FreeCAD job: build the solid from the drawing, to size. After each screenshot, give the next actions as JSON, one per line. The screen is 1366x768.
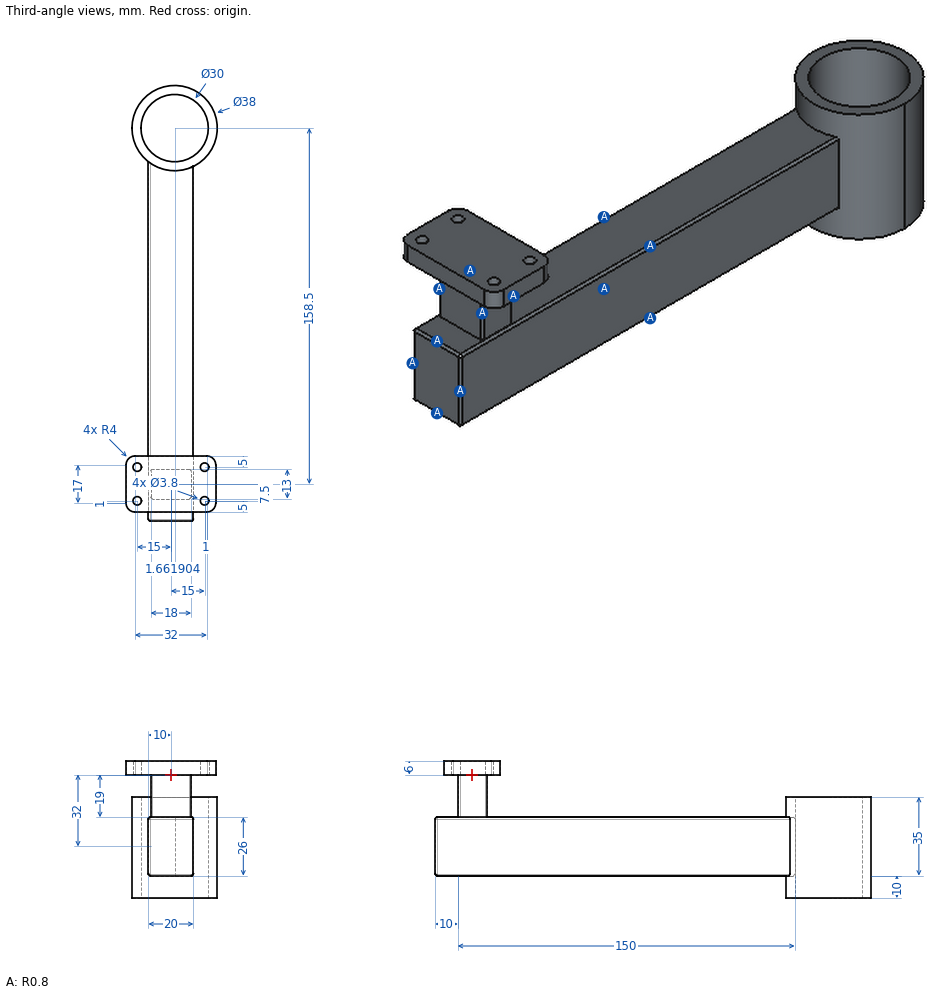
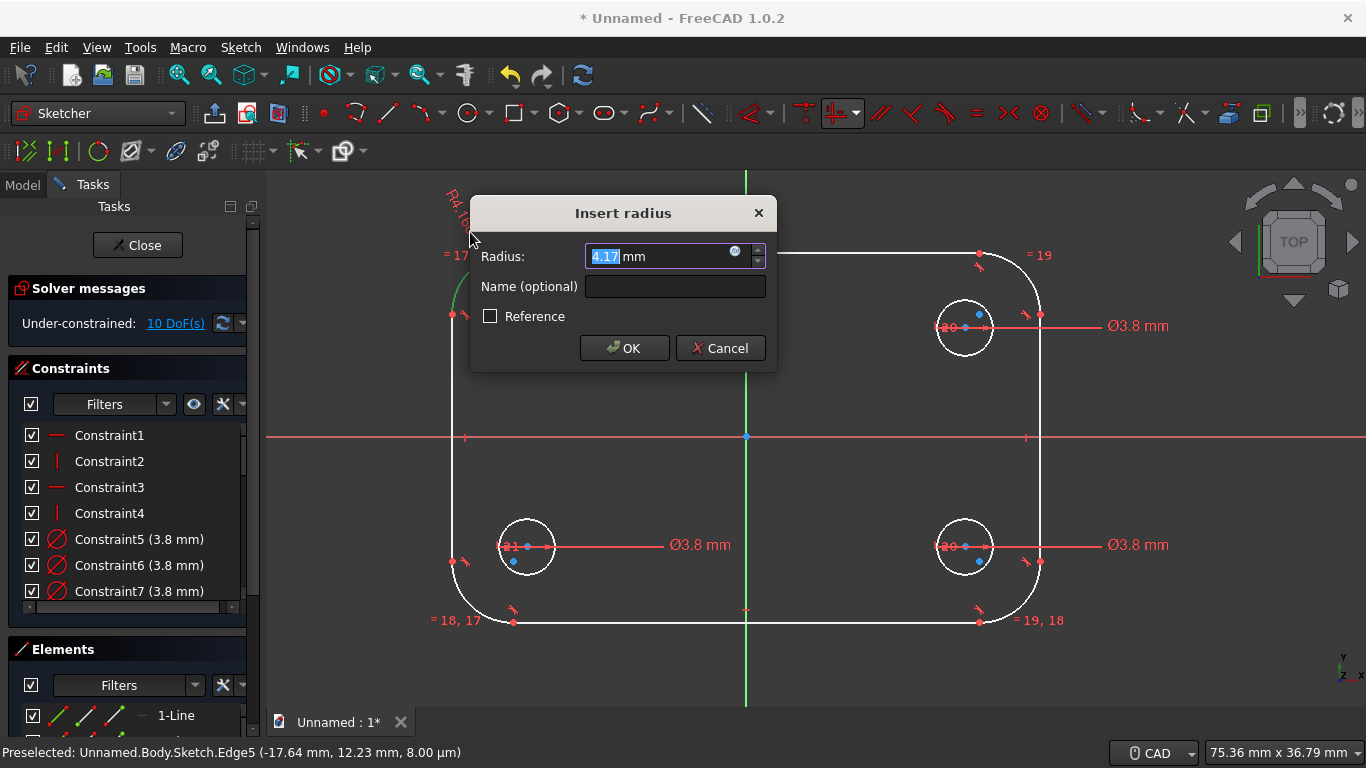
{"action": "type", "text": "4"}
{"action": "key", "text": "Return"}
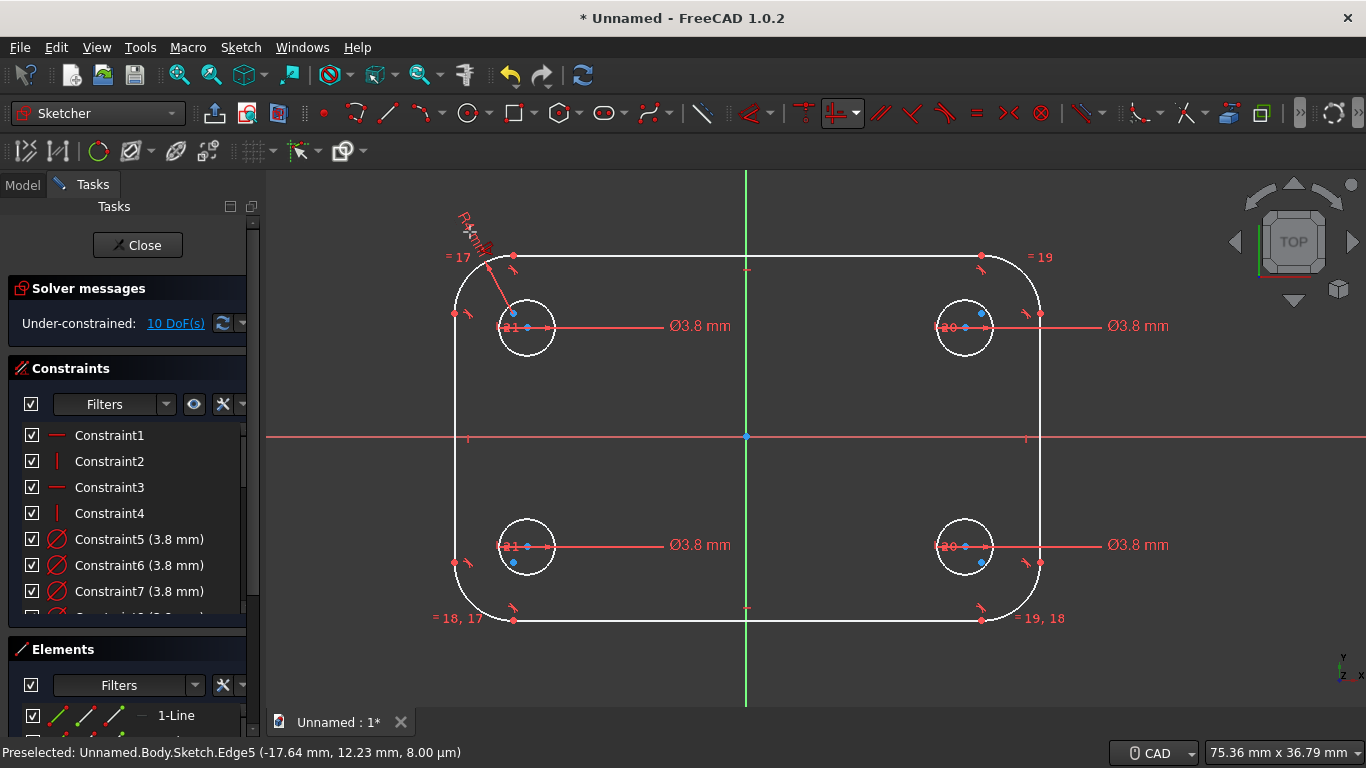
{"action": "left_click", "coordinate": [841, 256]}
{"action": "left_click", "coordinate": [640, 222]}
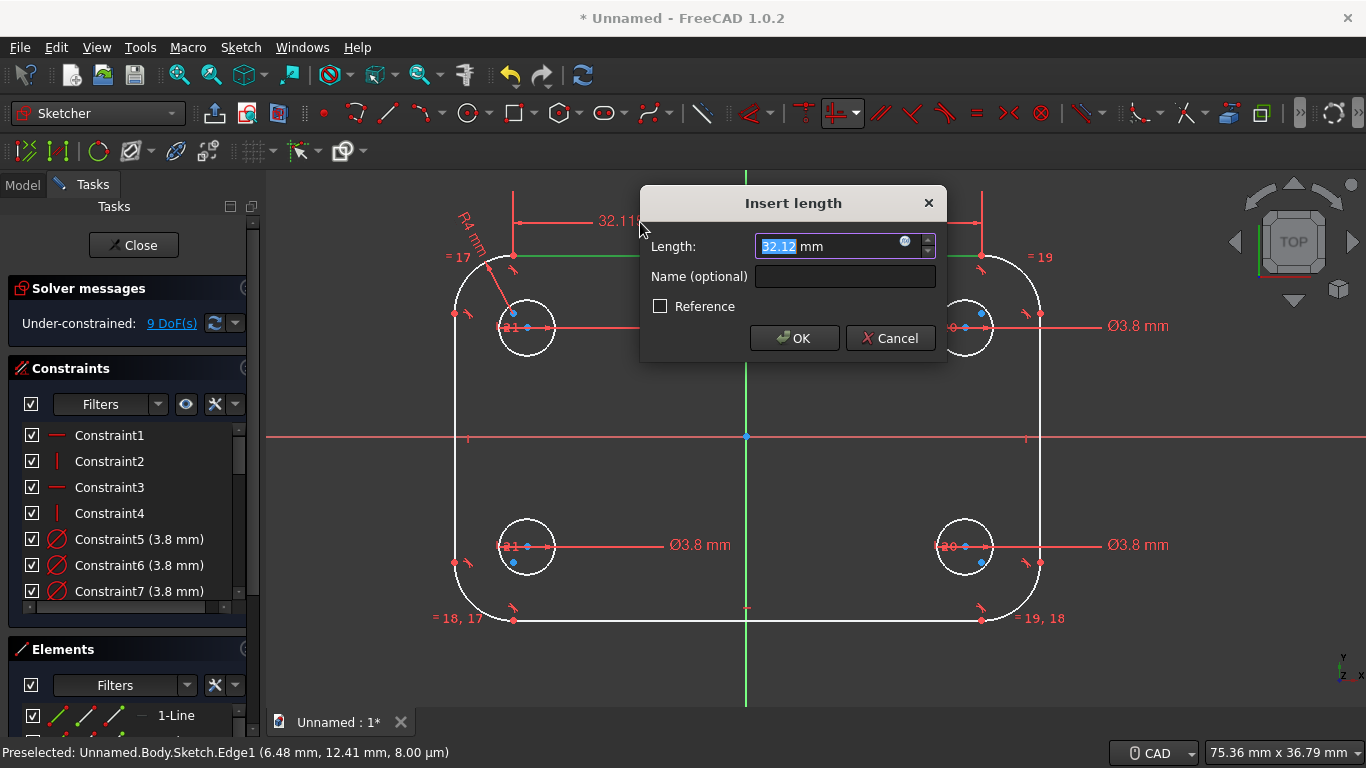
{"action": "type", "text": "32"}
{"action": "key", "text": "Return"}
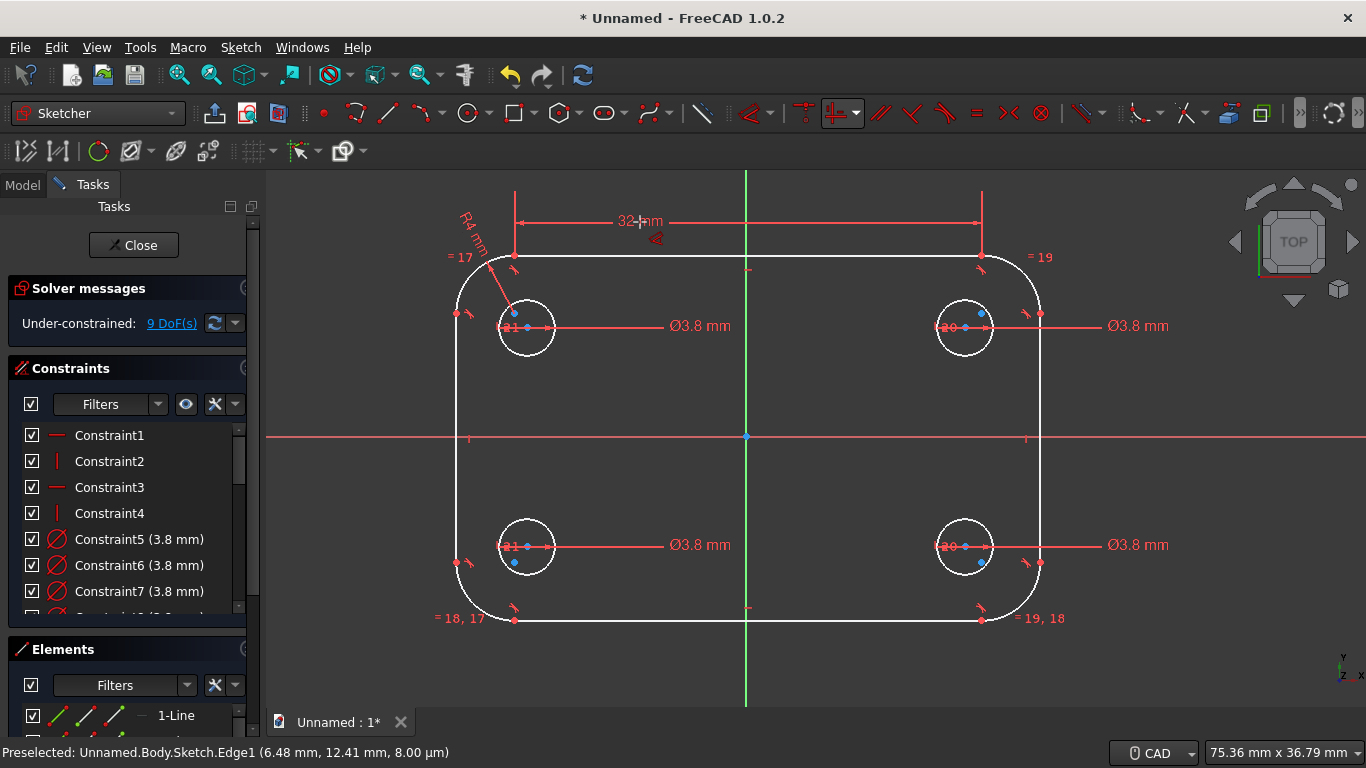
{"action": "left_click", "coordinate": [456, 389]}
{"action": "left_click", "coordinate": [422, 381]}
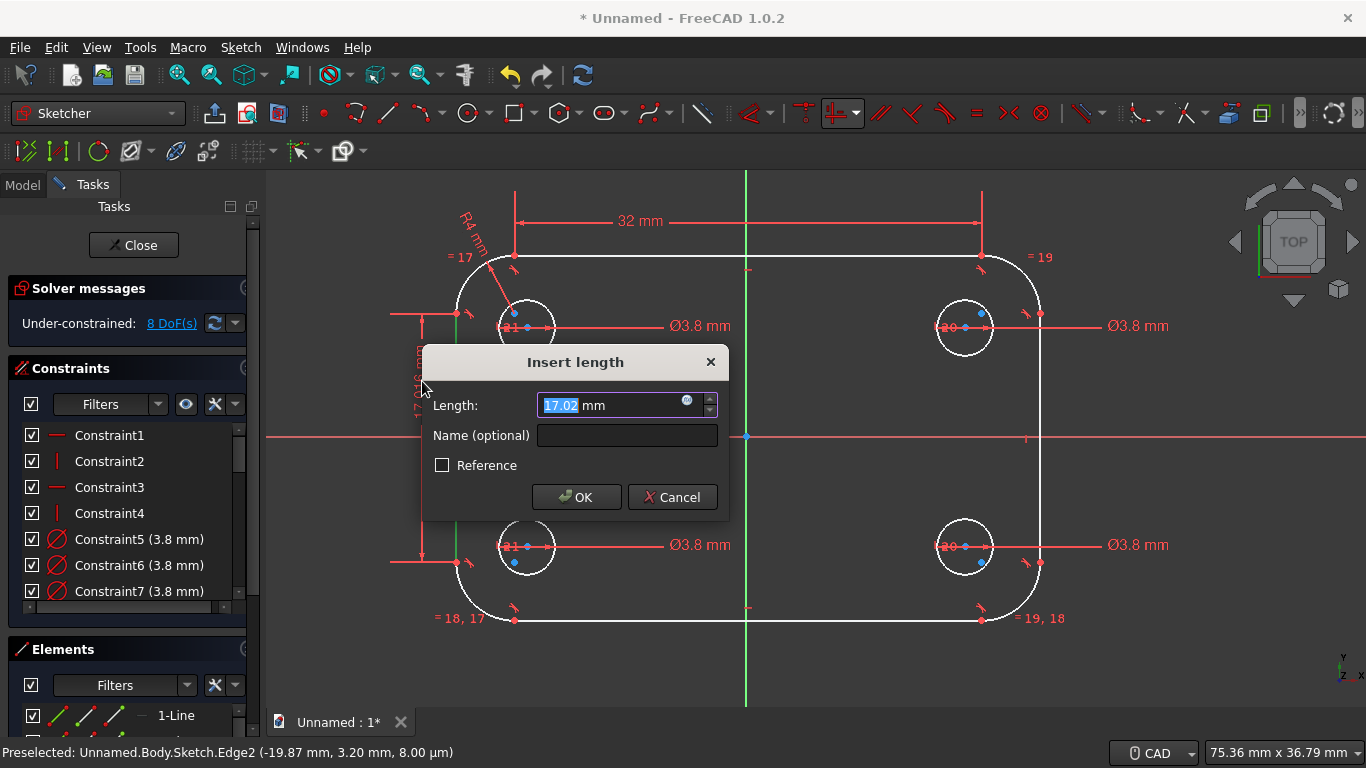
{"action": "type", "text": "17"}
{"action": "key", "text": "Return"}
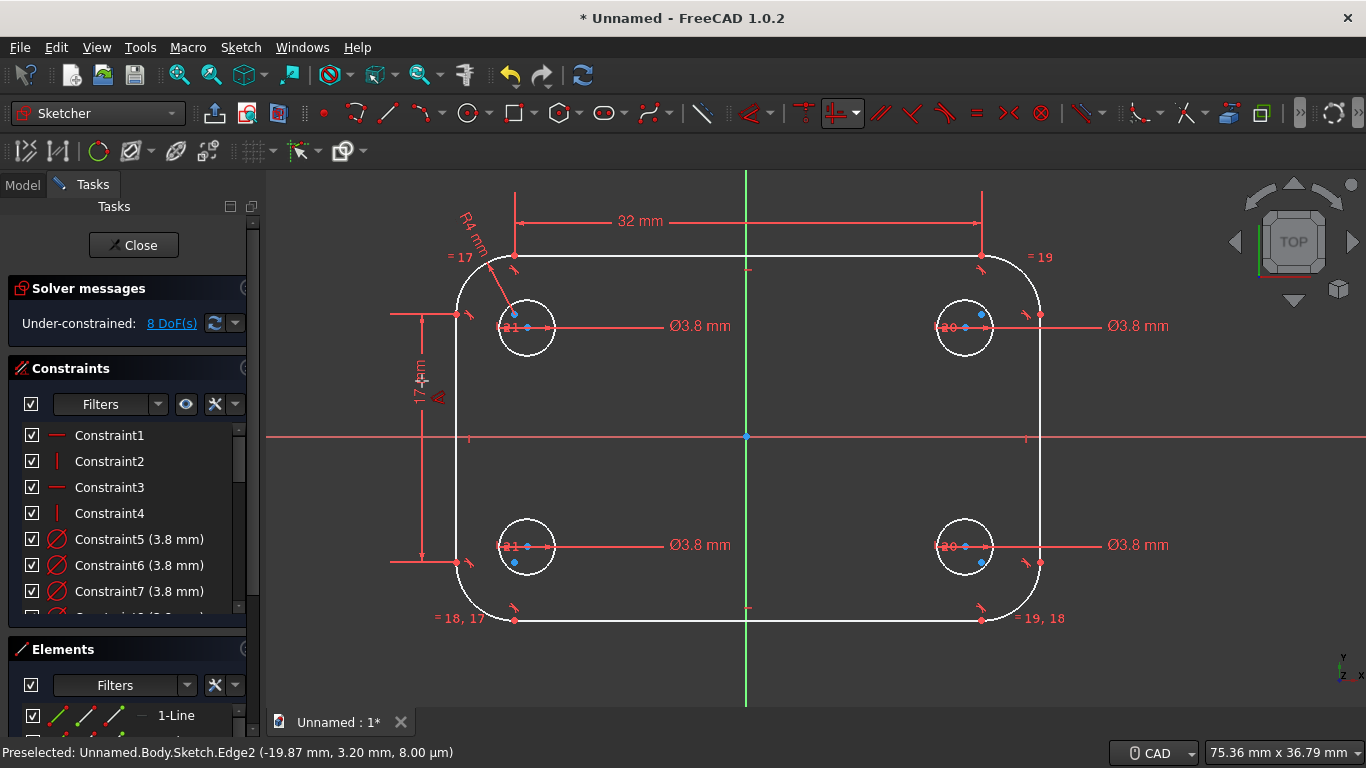
{"action": "left_click", "coordinate": [965, 547]}
{"action": "left_click", "coordinate": [856, 581]}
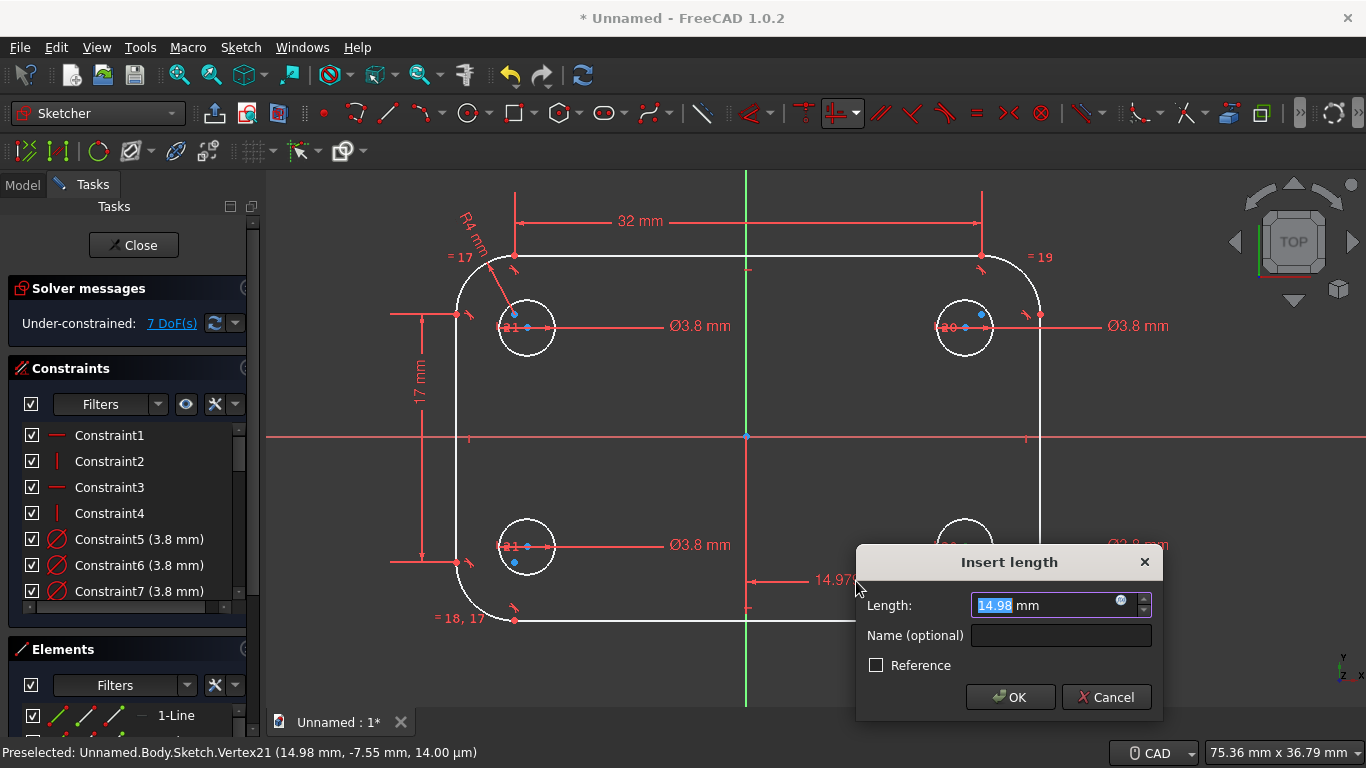
{"action": "type", "text": "15"}
{"action": "key", "text": "Return"}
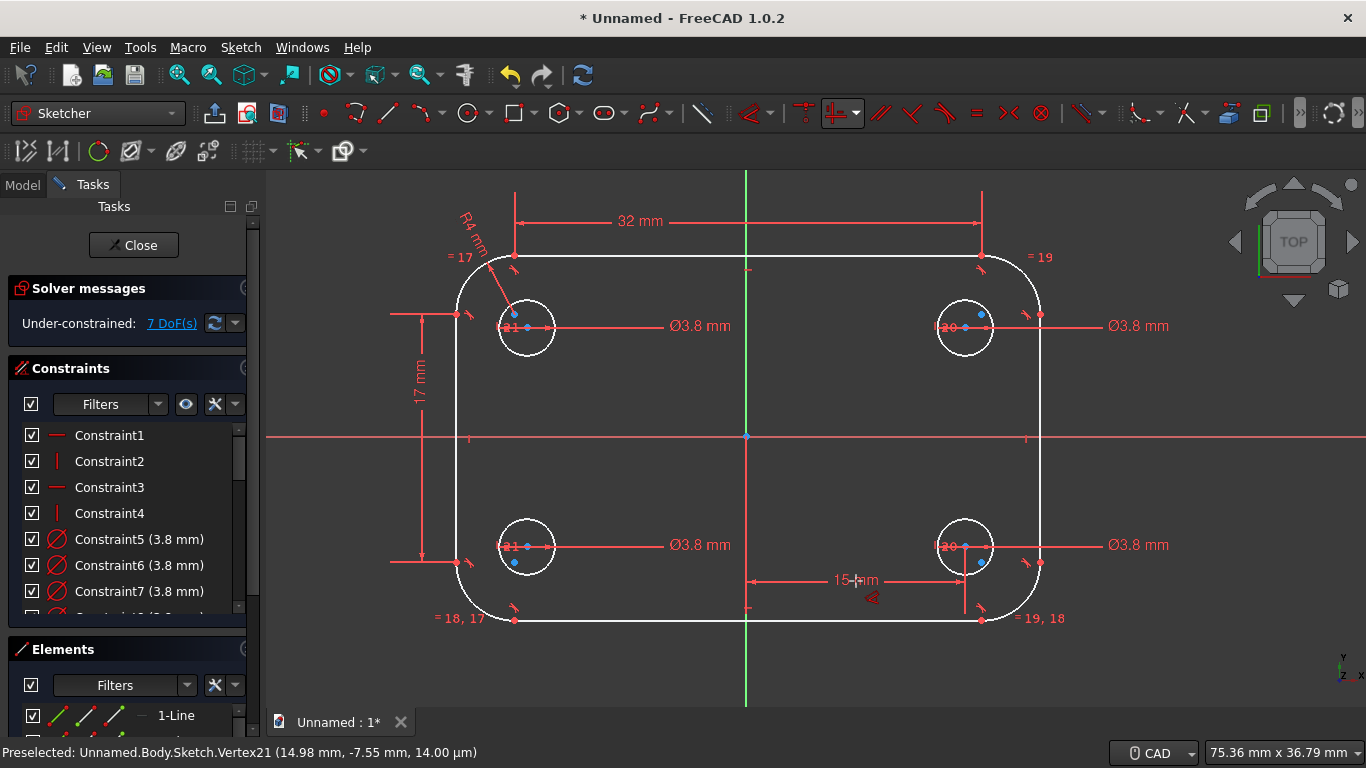
{"action": "left_click", "coordinate": [527, 547]}
{"action": "left_click", "coordinate": [637, 581]}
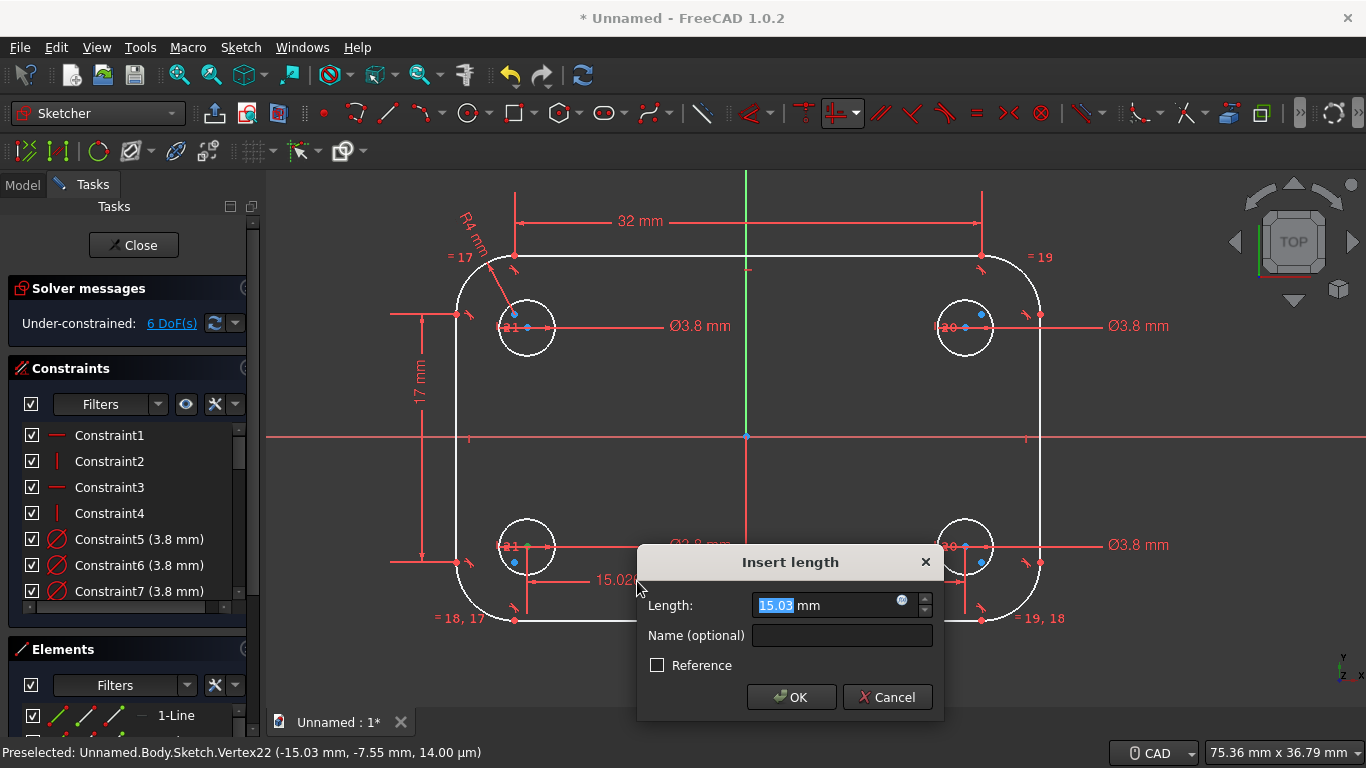
{"action": "type", "text": "15"}
{"action": "key", "text": "Return"}